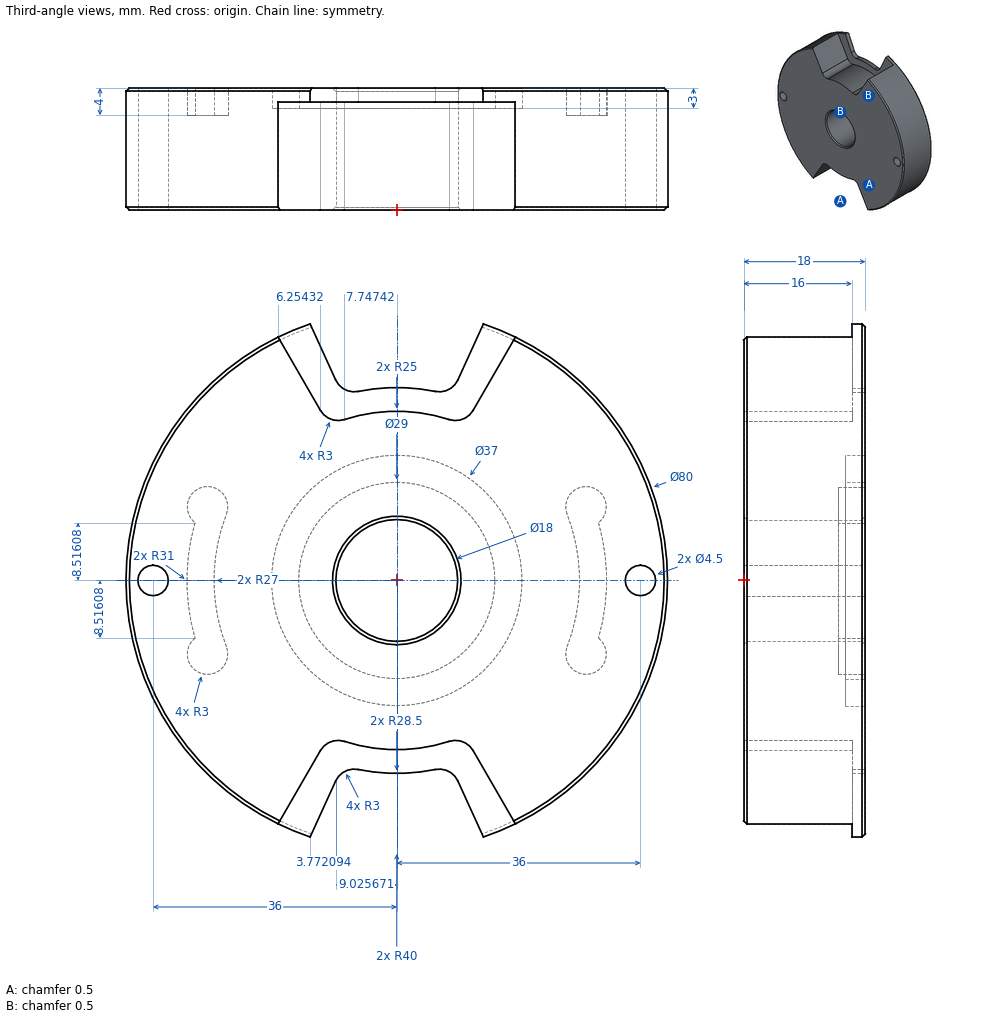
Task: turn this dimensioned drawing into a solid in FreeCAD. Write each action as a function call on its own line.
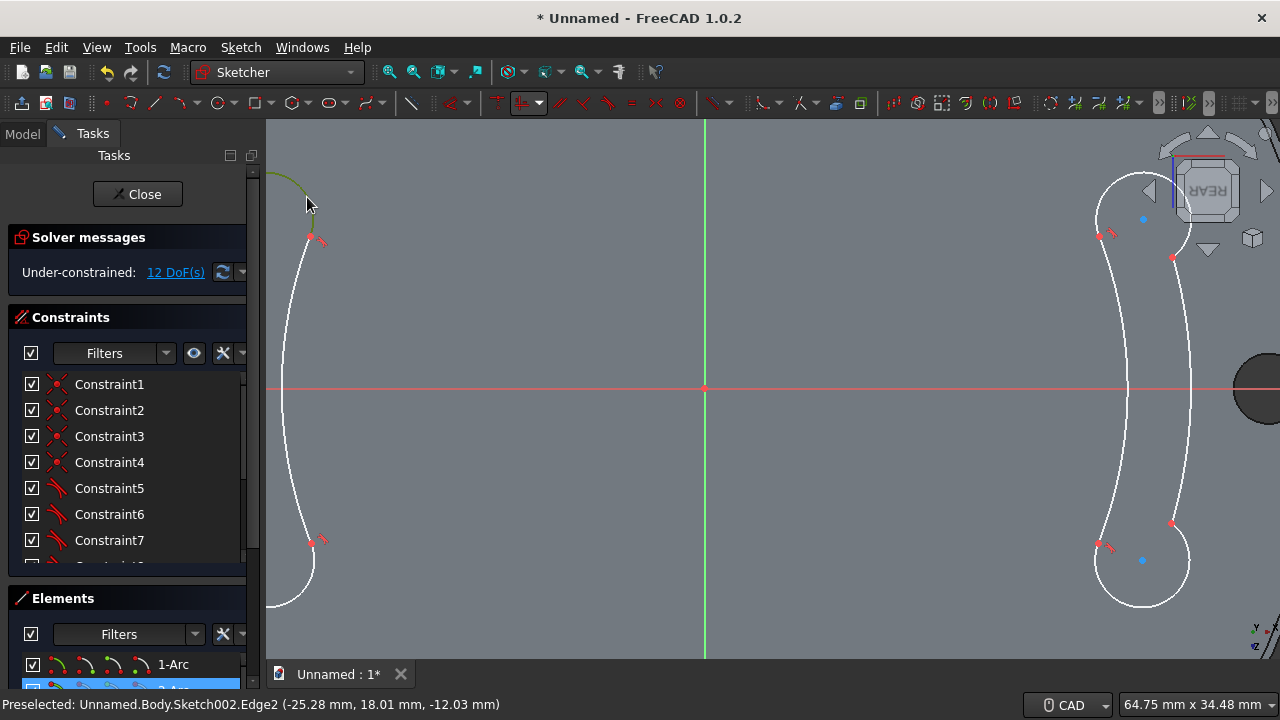
click(295, 598)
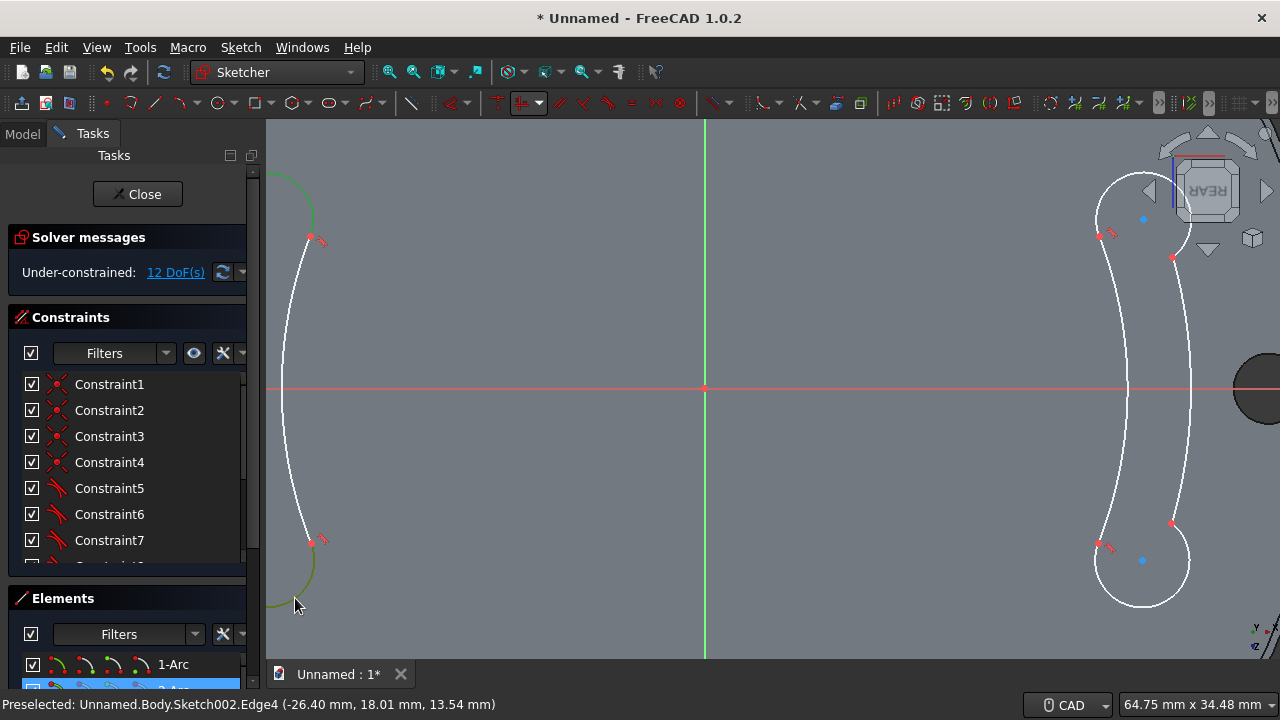
click(1115, 599)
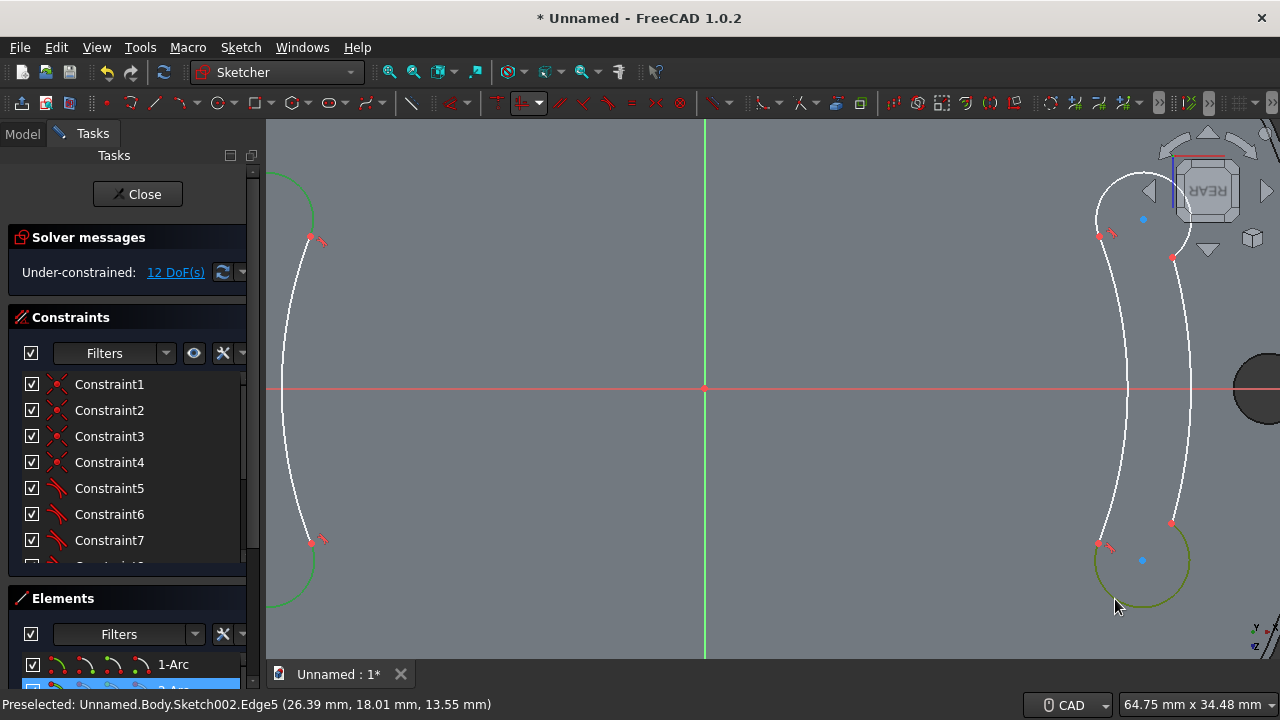
click(1102, 196)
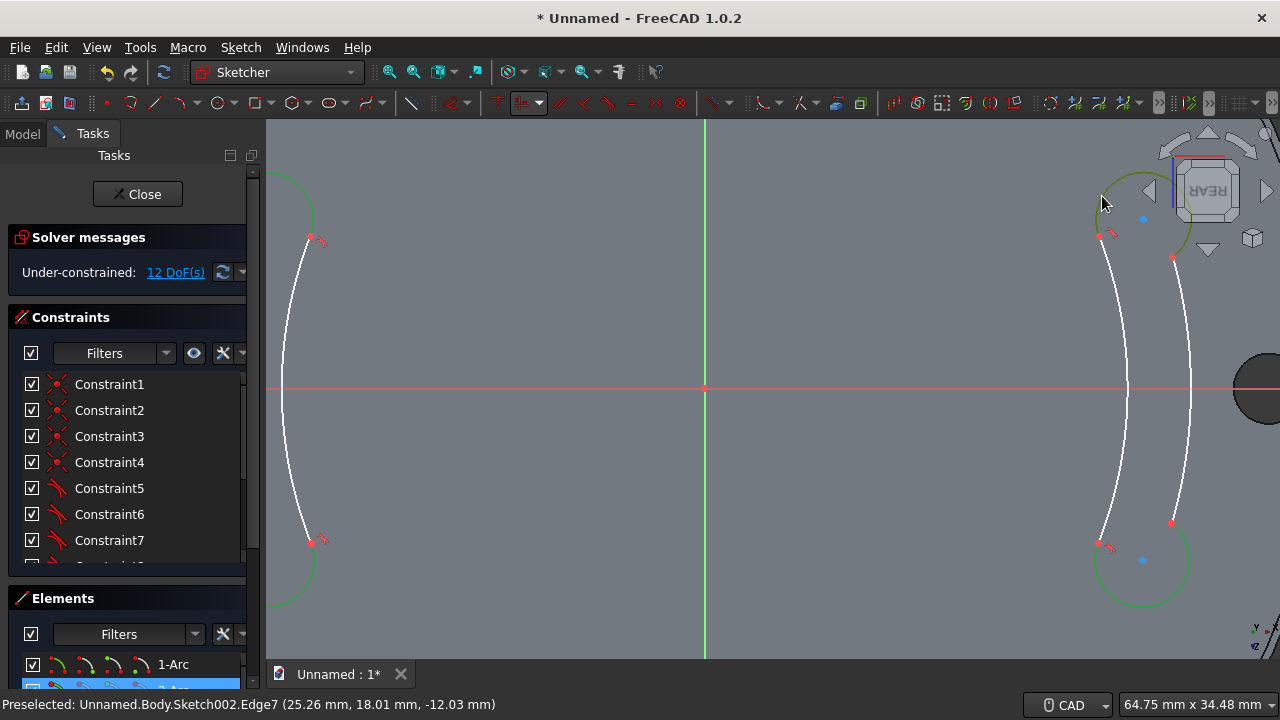
click(632, 104)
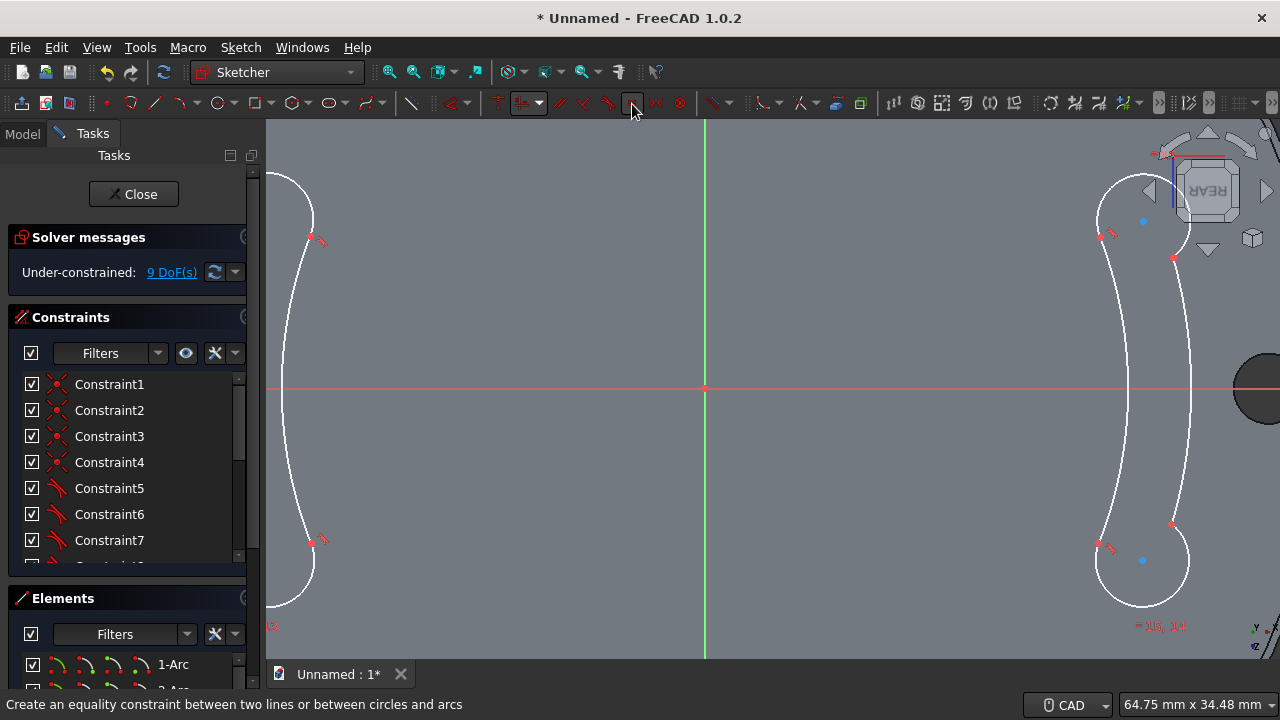
scroll(704, 389, down, 3)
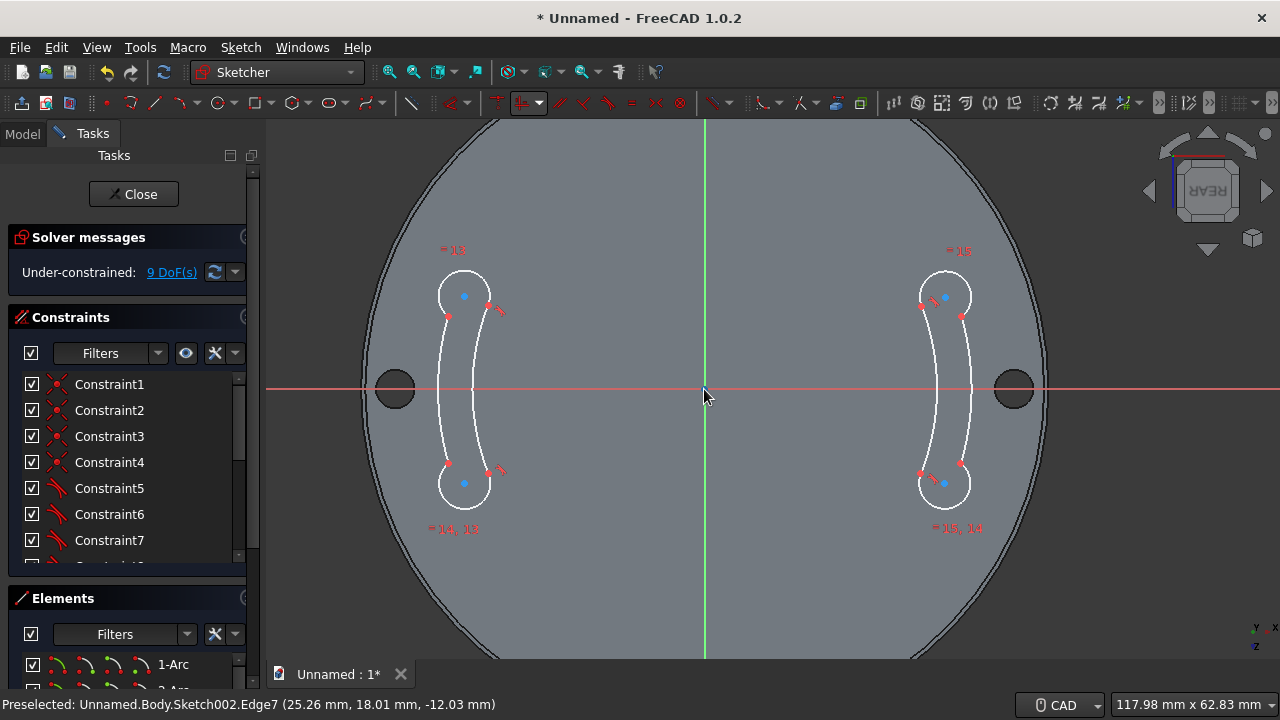
click(440, 360)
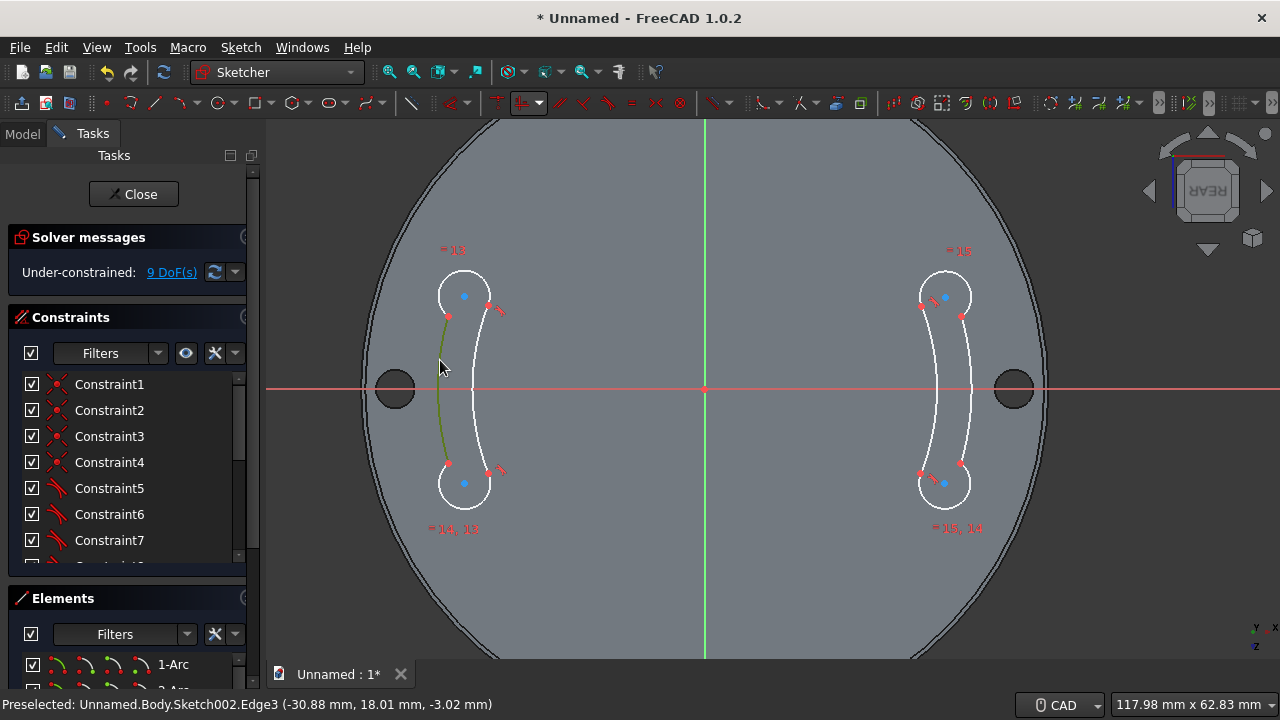
click(970, 420)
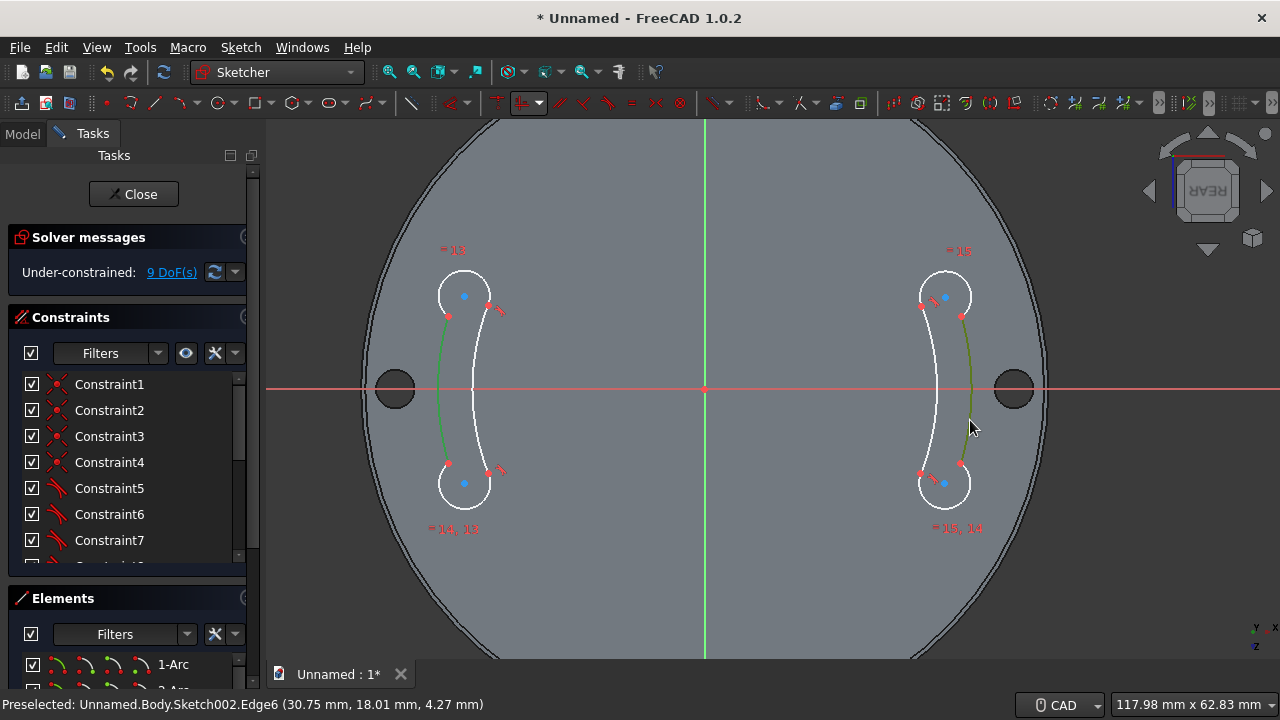
click(632, 104)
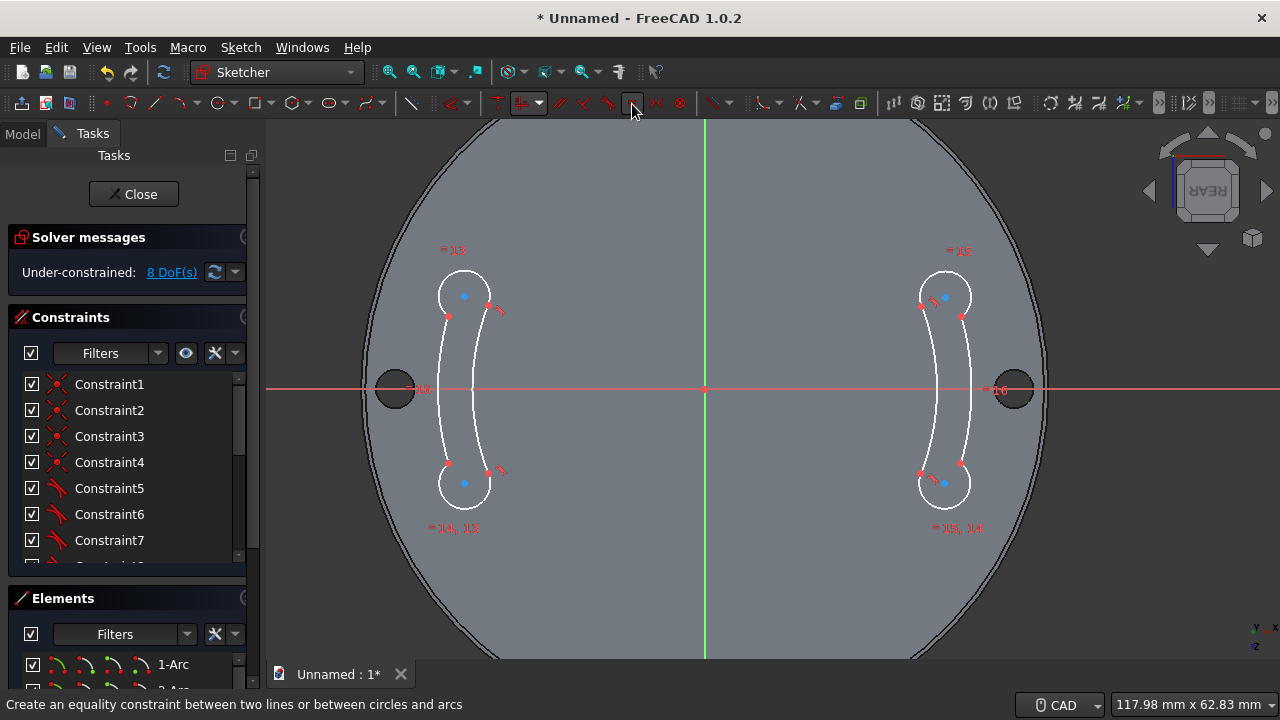
click(475, 355)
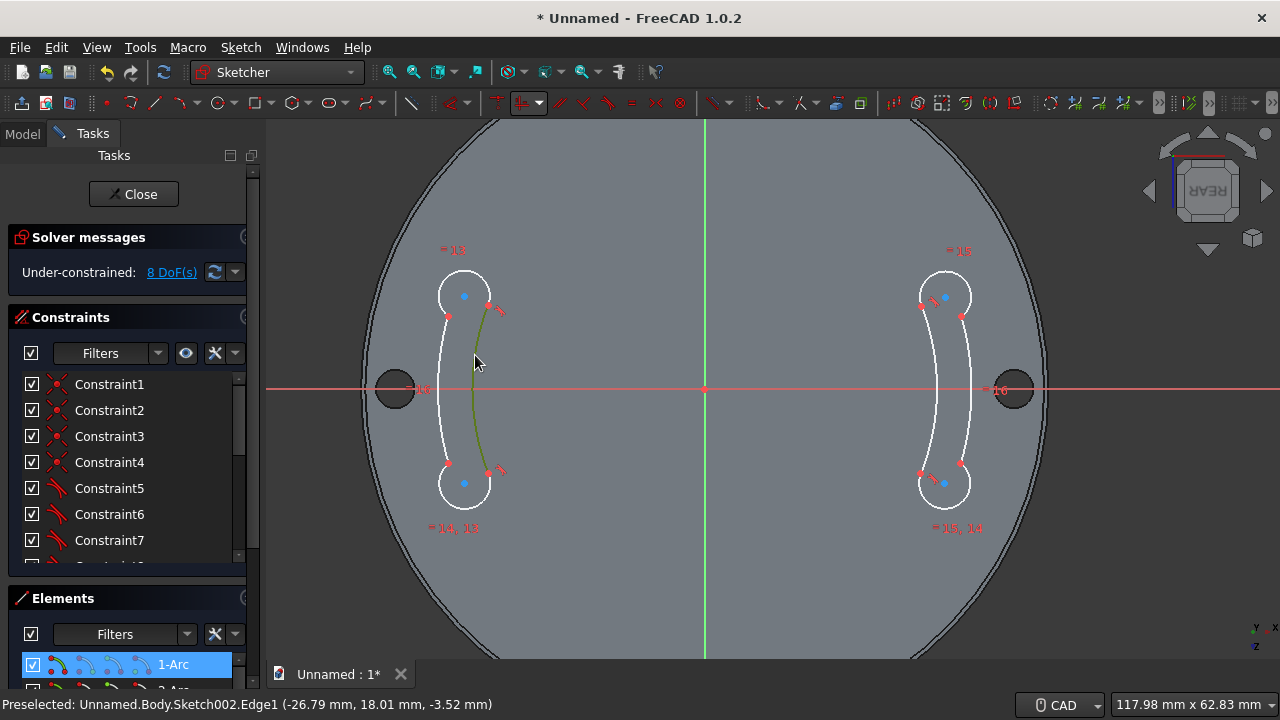
click(934, 424)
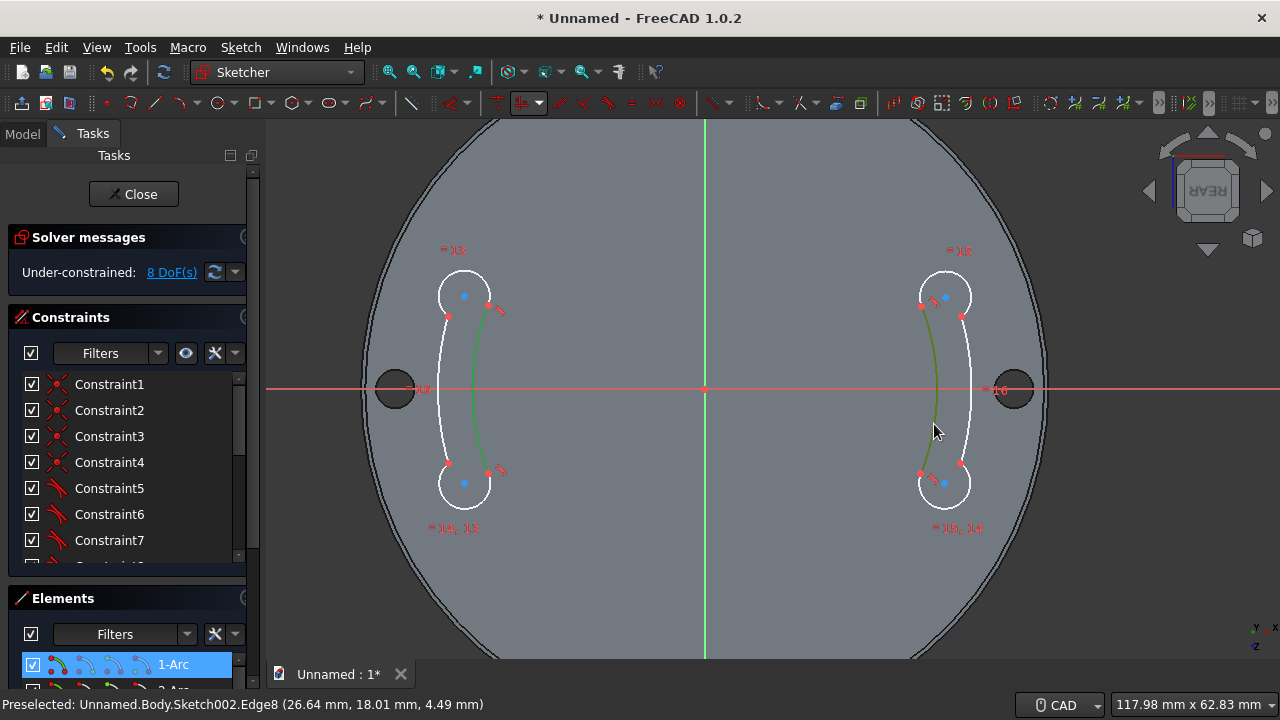
click(632, 104)